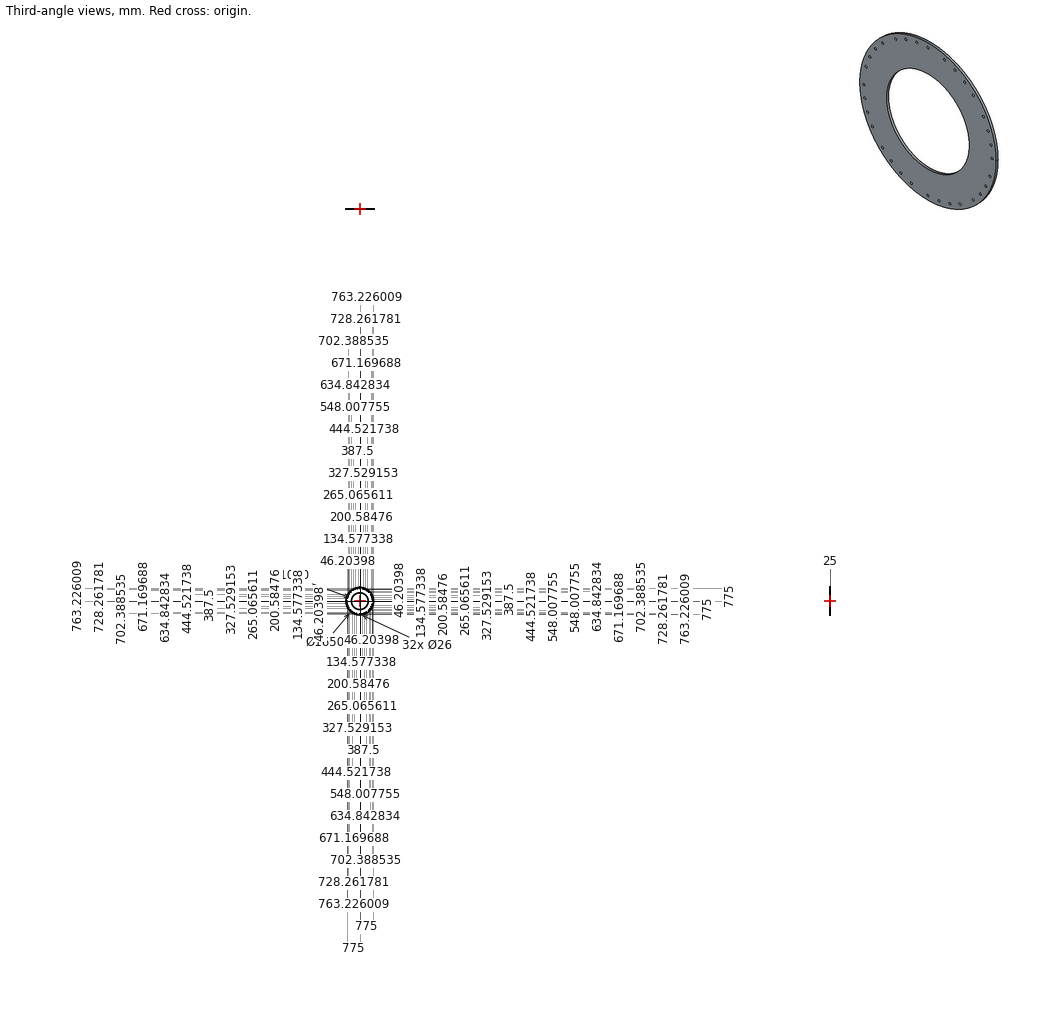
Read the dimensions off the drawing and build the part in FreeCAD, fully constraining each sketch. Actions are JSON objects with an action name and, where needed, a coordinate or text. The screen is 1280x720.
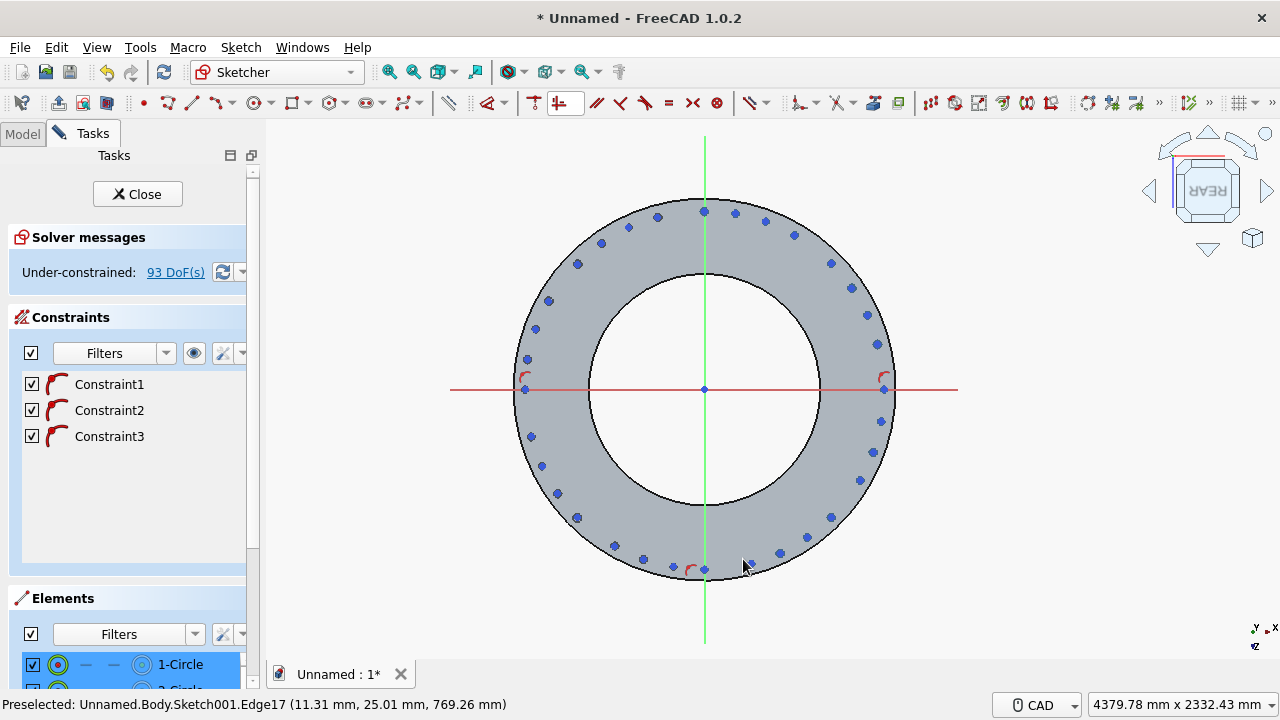
{"action": "scroll", "coordinate": [676, 565], "scroll_direction": "up", "scroll_amount": 8}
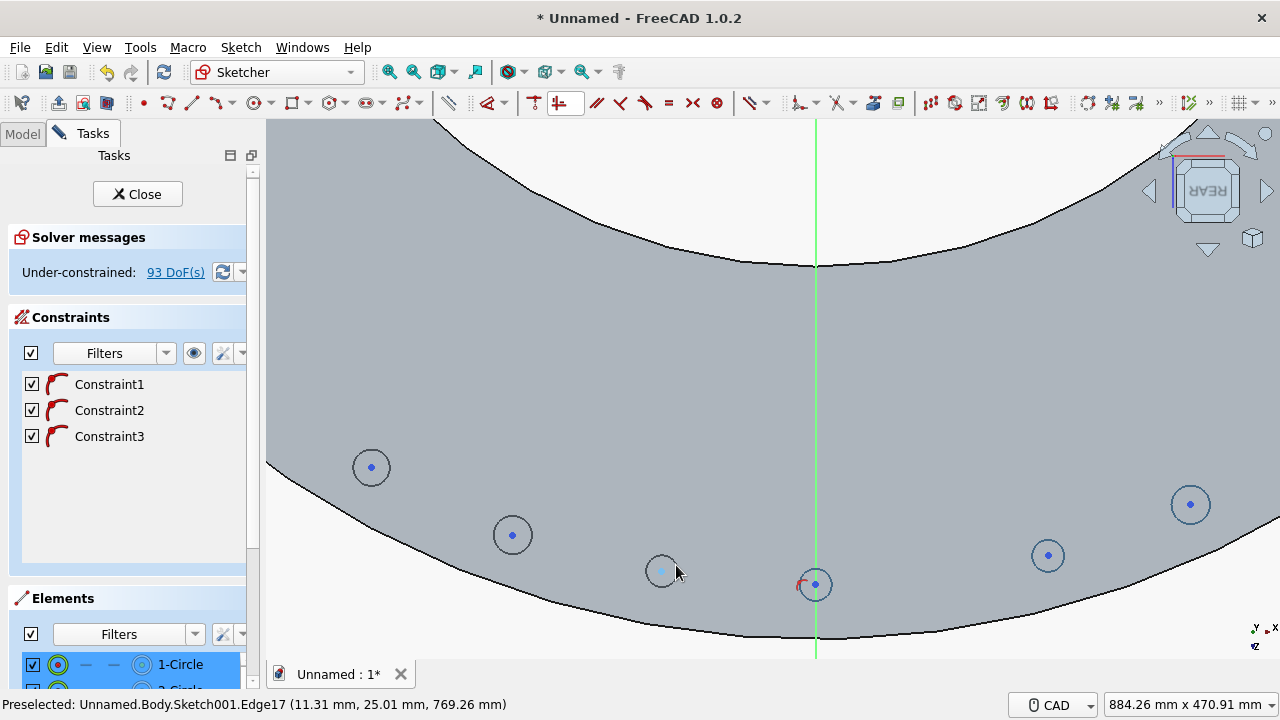
{"action": "left_click", "coordinate": [673, 560]}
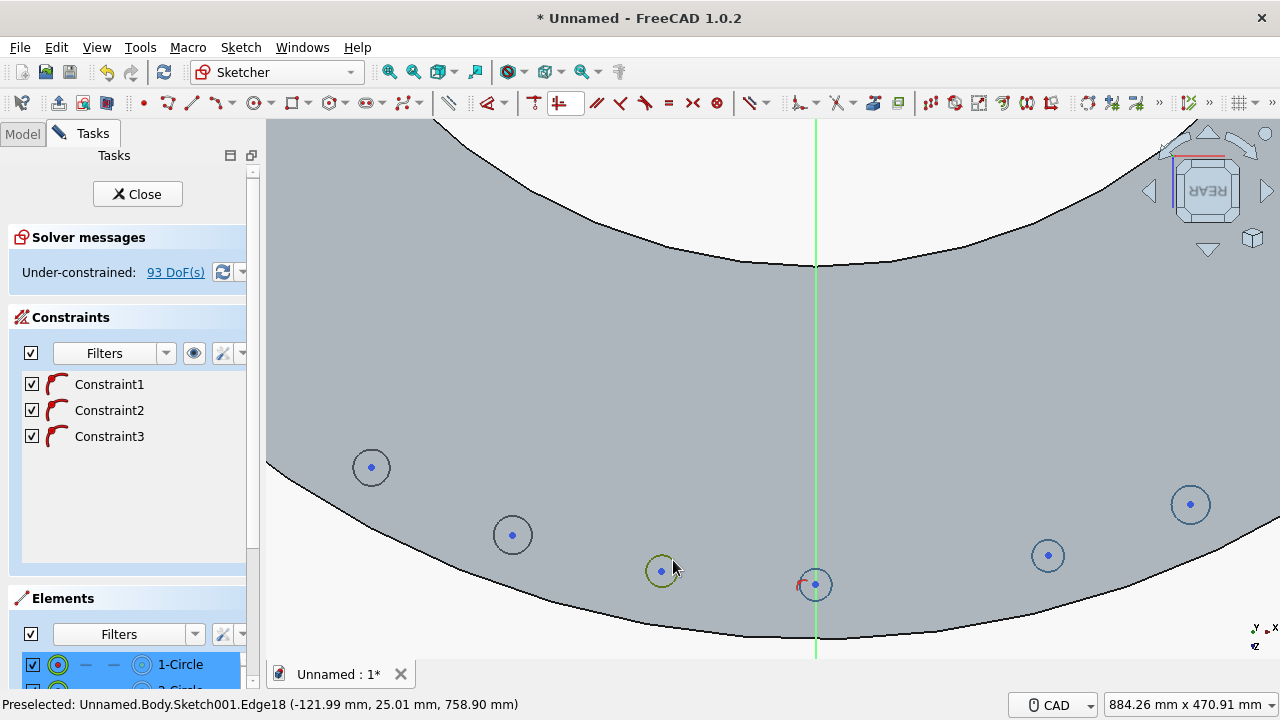
{"action": "left_click", "coordinate": [526, 521]}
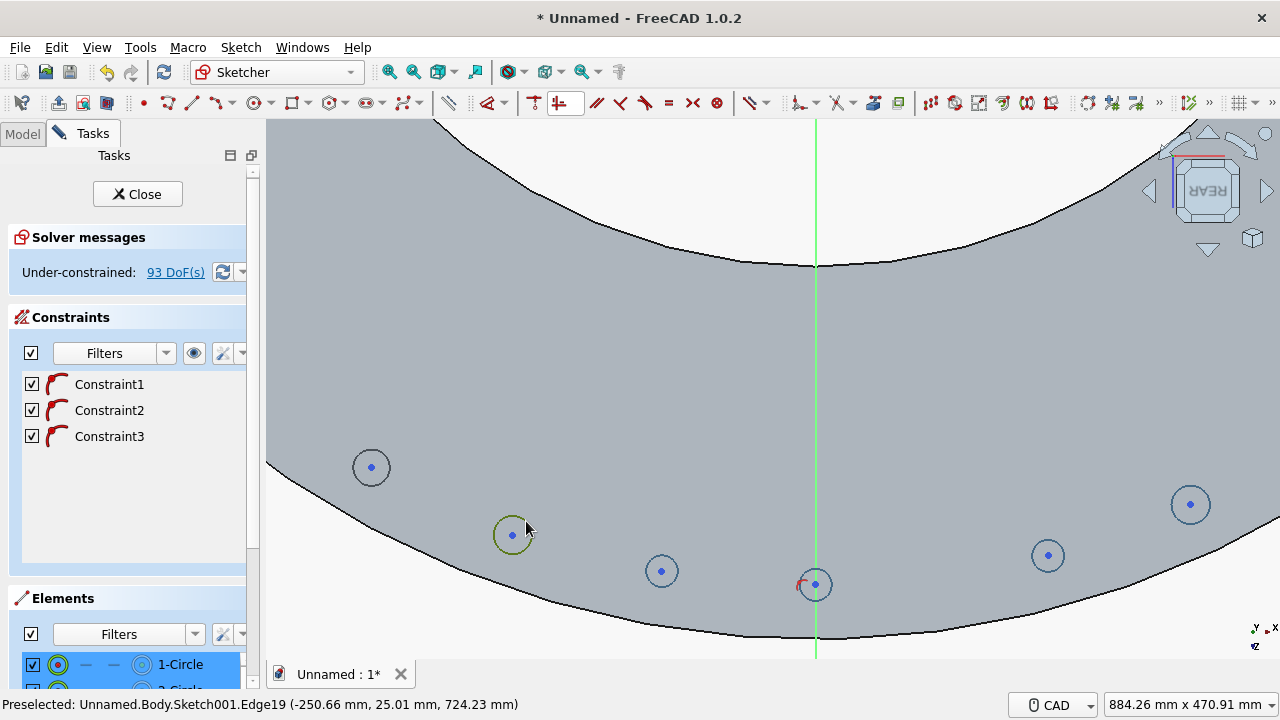
{"action": "left_click", "coordinate": [384, 455]}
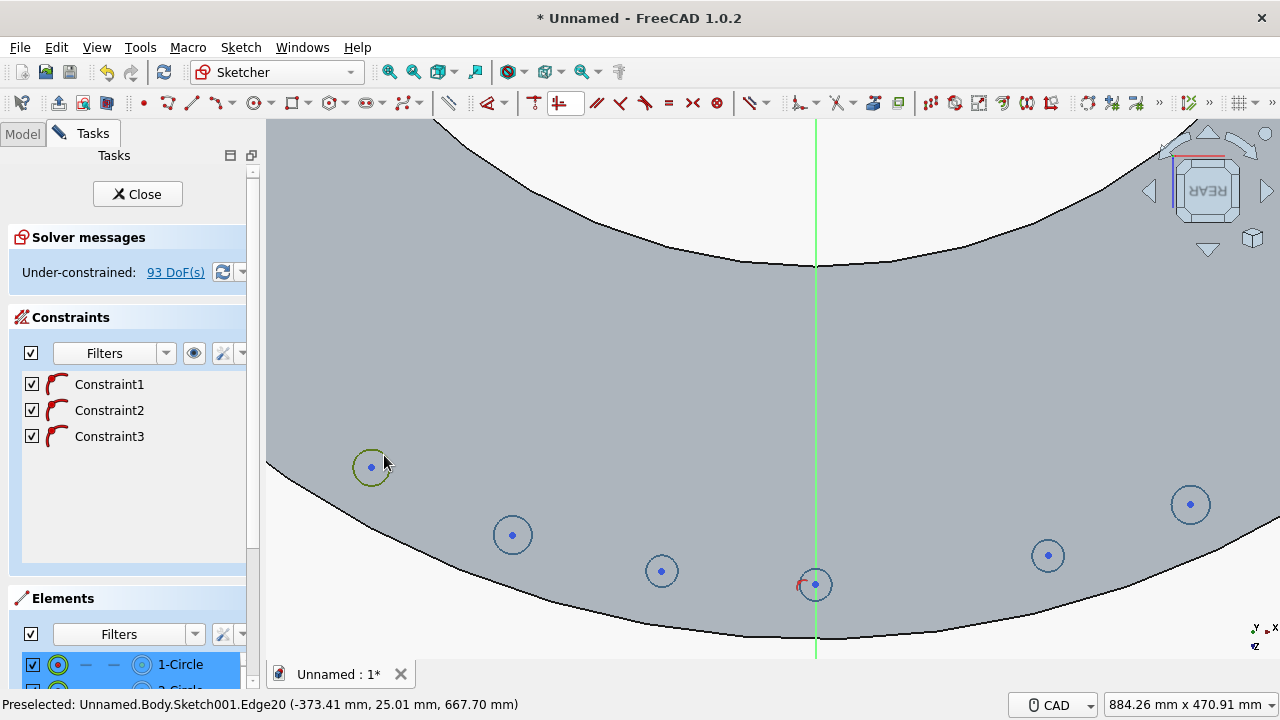
{"action": "scroll", "coordinate": [676, 565], "scroll_direction": "down", "scroll_amount": 8}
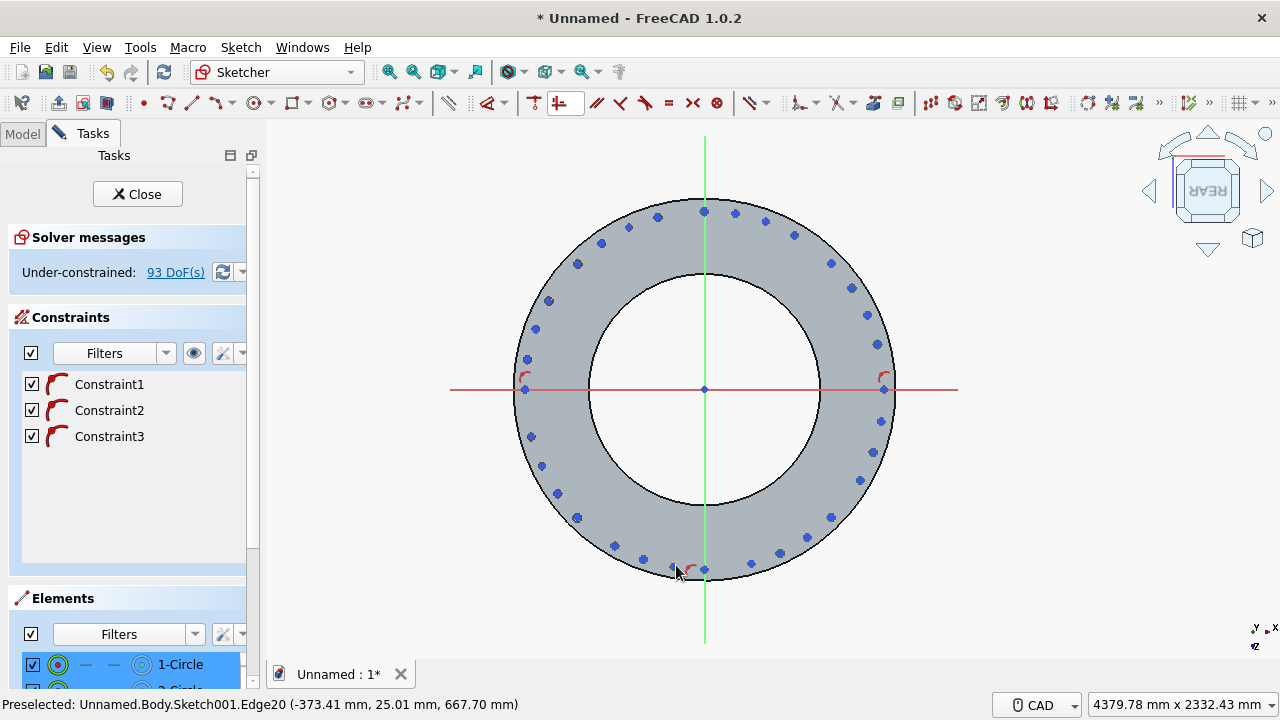
{"action": "scroll", "coordinate": [580, 515], "scroll_direction": "up", "scroll_amount": 6}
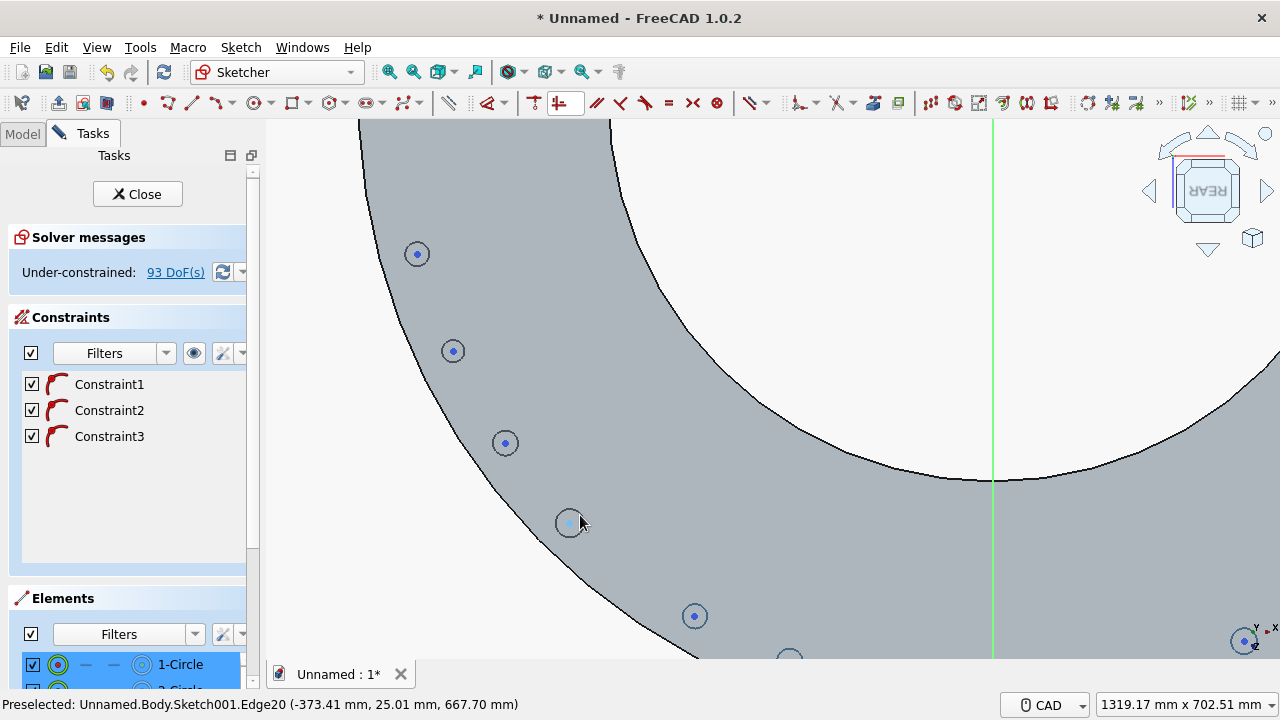
{"action": "left_click", "coordinate": [580, 513]}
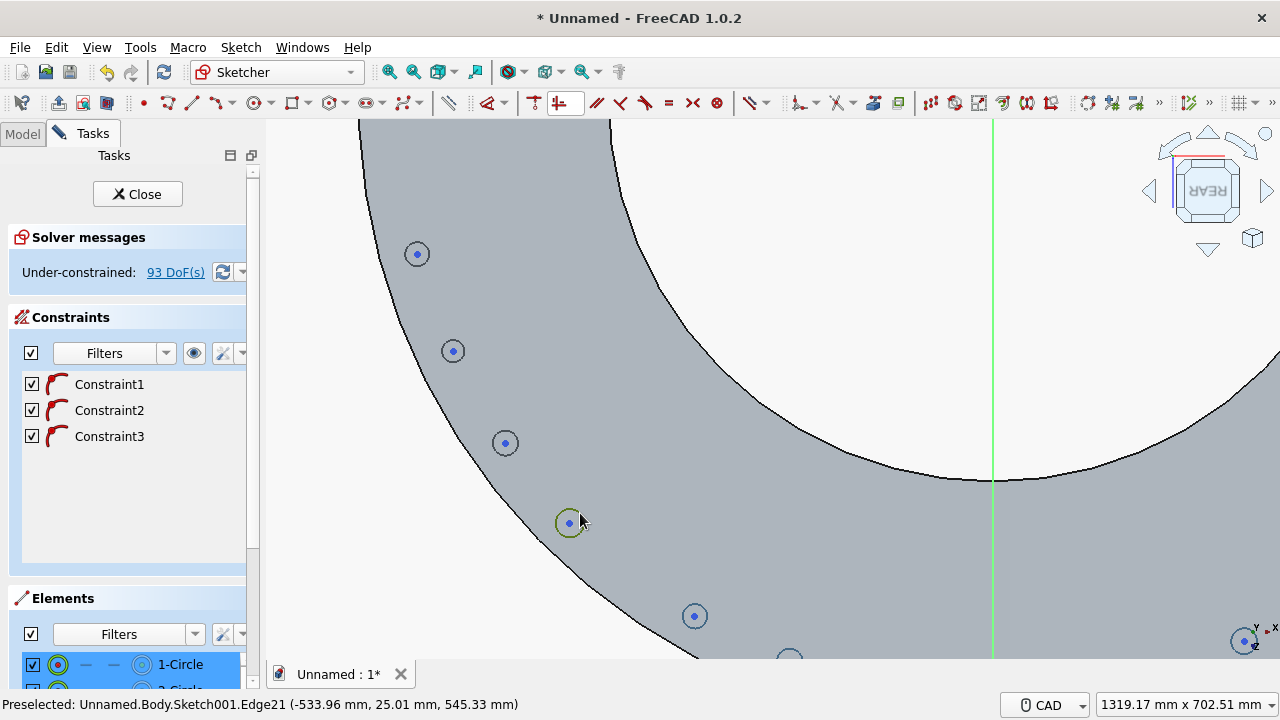
{"action": "left_click", "coordinate": [514, 434]}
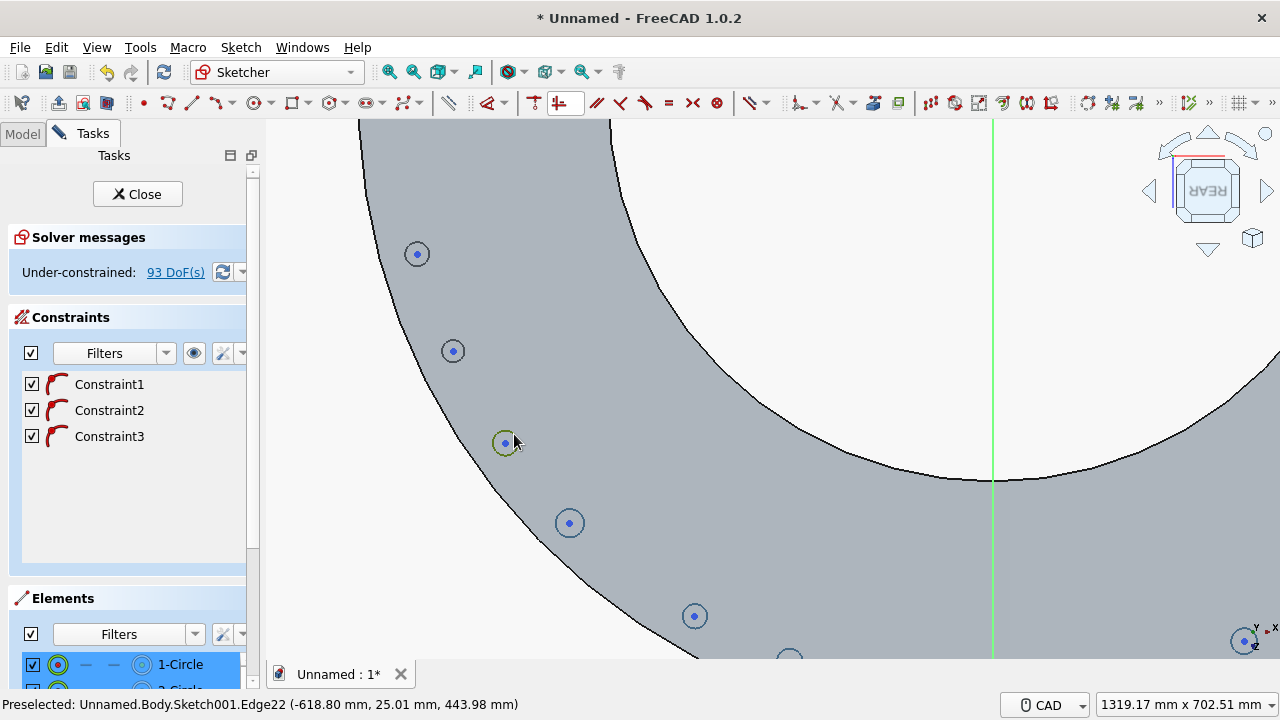
{"action": "scroll", "coordinate": [461, 343], "scroll_direction": "up", "scroll_amount": 2}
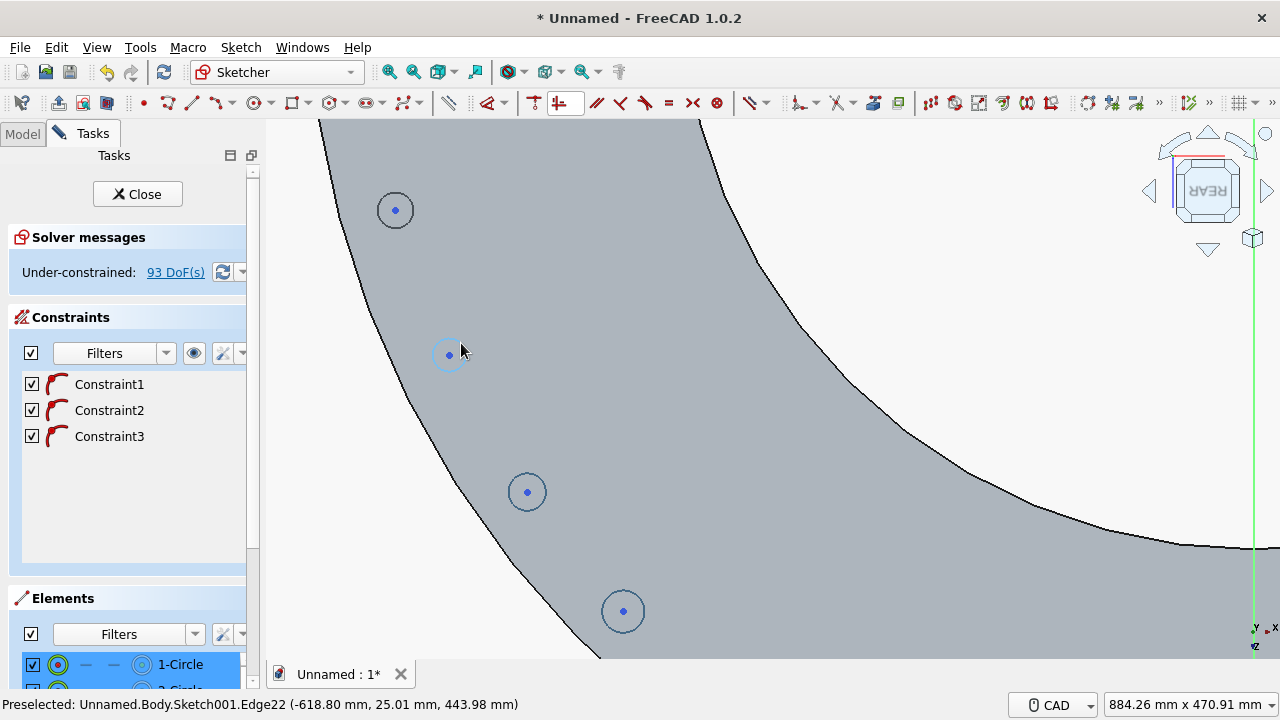
{"action": "left_click", "coordinate": [461, 343]}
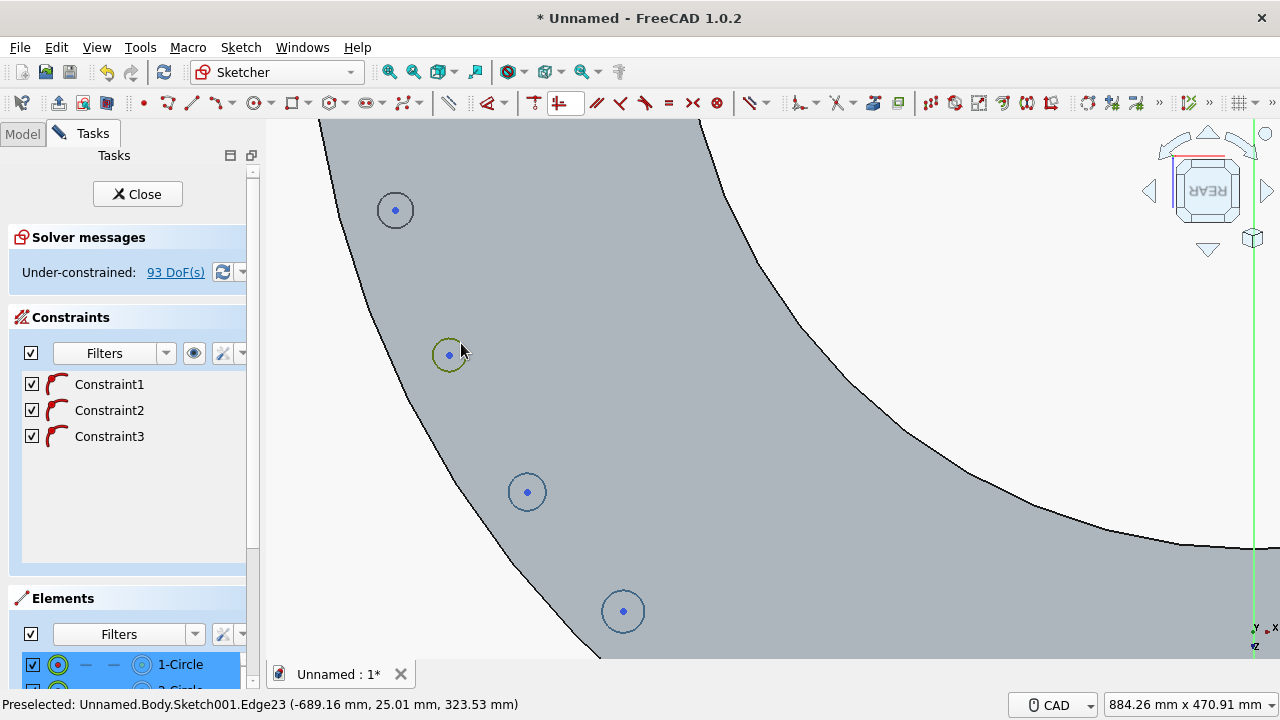
{"action": "left_click", "coordinate": [408, 198]}